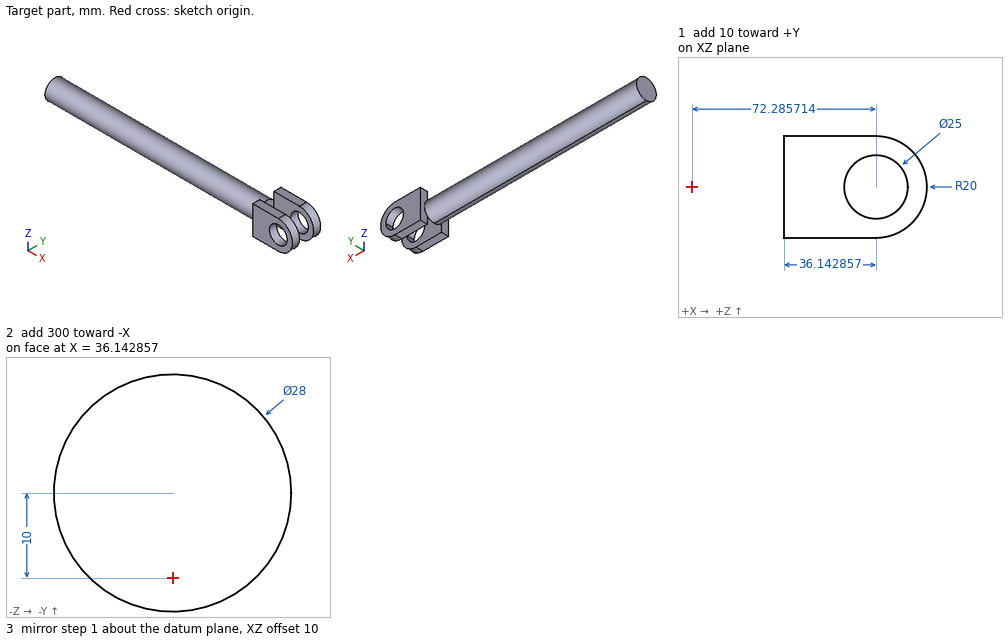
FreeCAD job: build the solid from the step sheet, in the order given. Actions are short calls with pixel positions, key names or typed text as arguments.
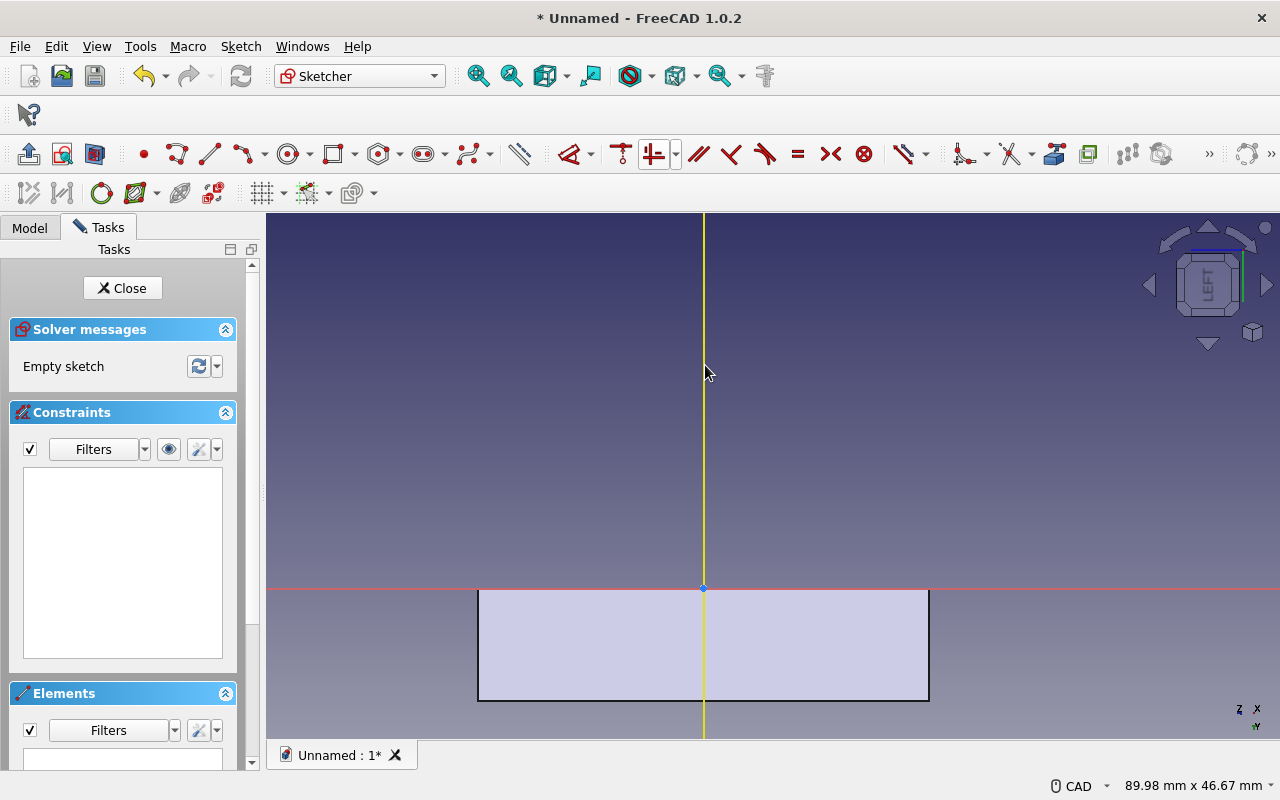
click(288, 154)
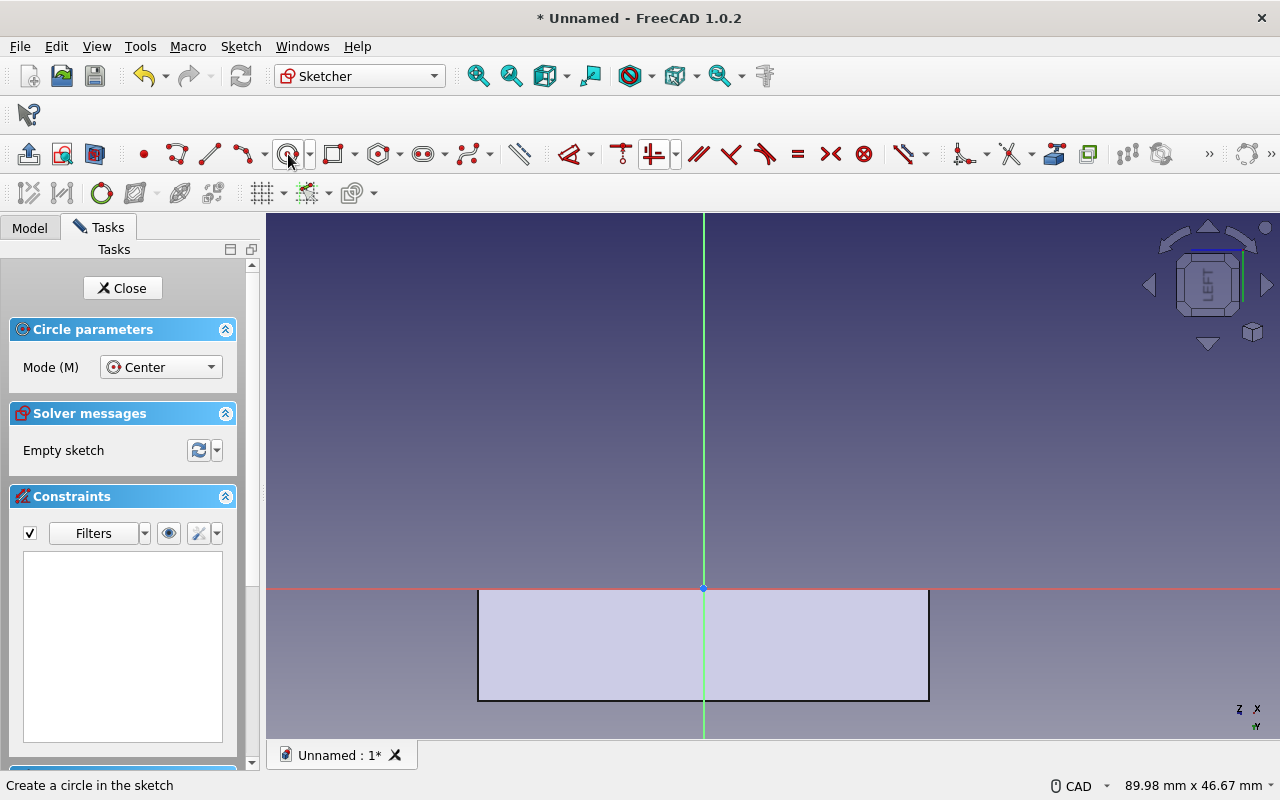
click(704, 476)
move(815, 364)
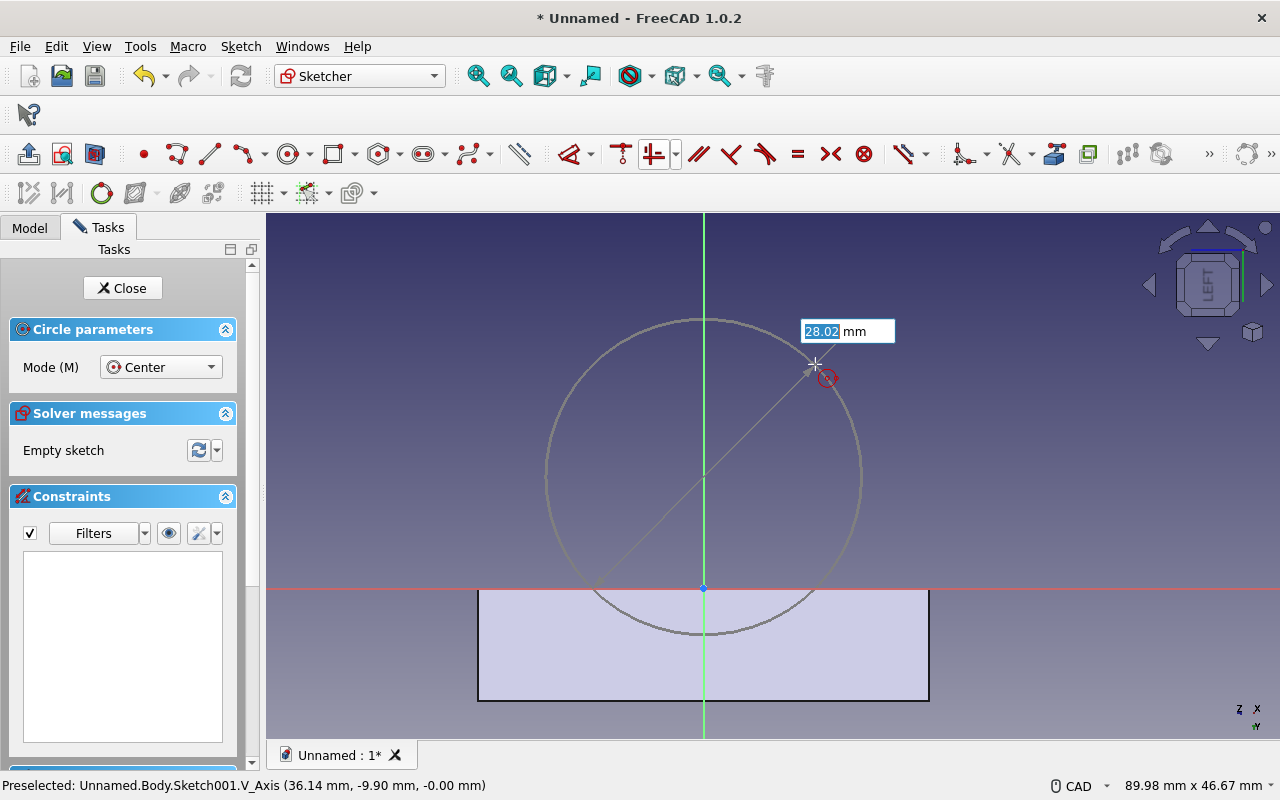
text(28)
key(Return)
key(Escape)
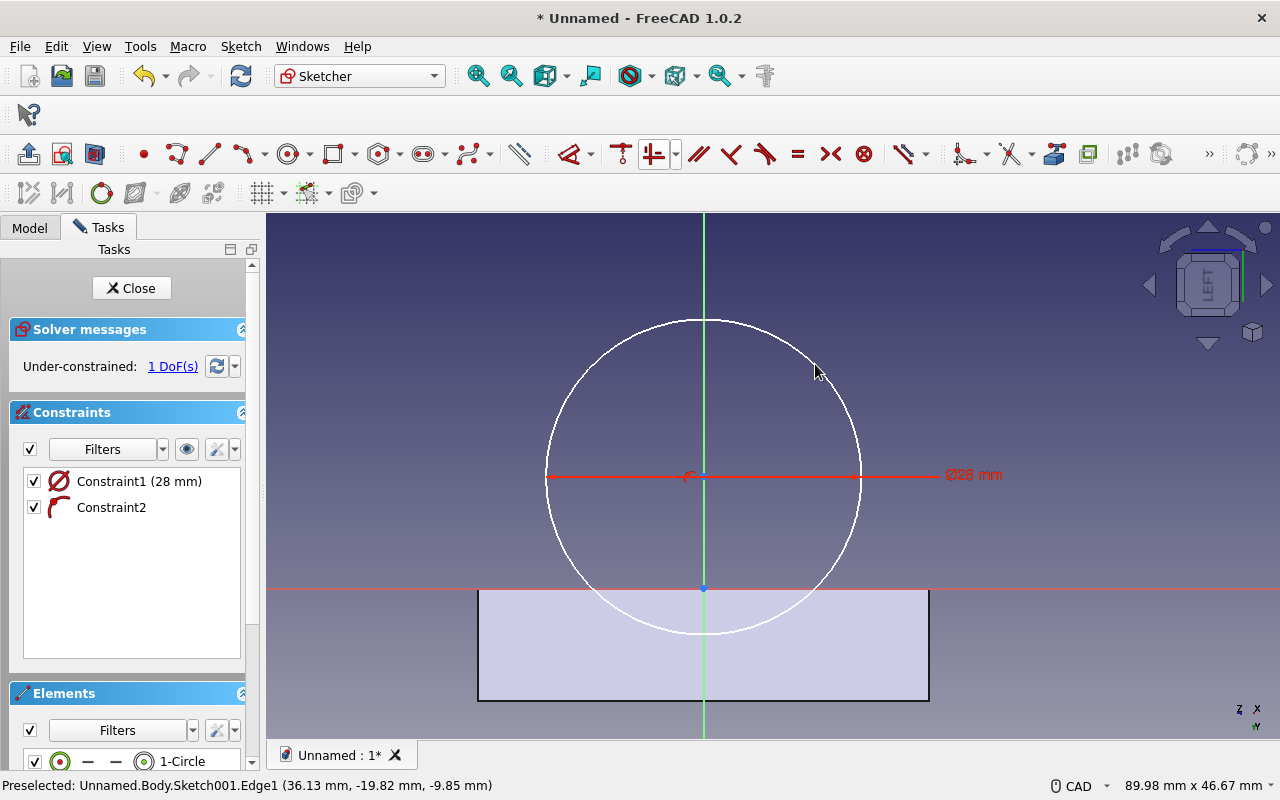
key(d)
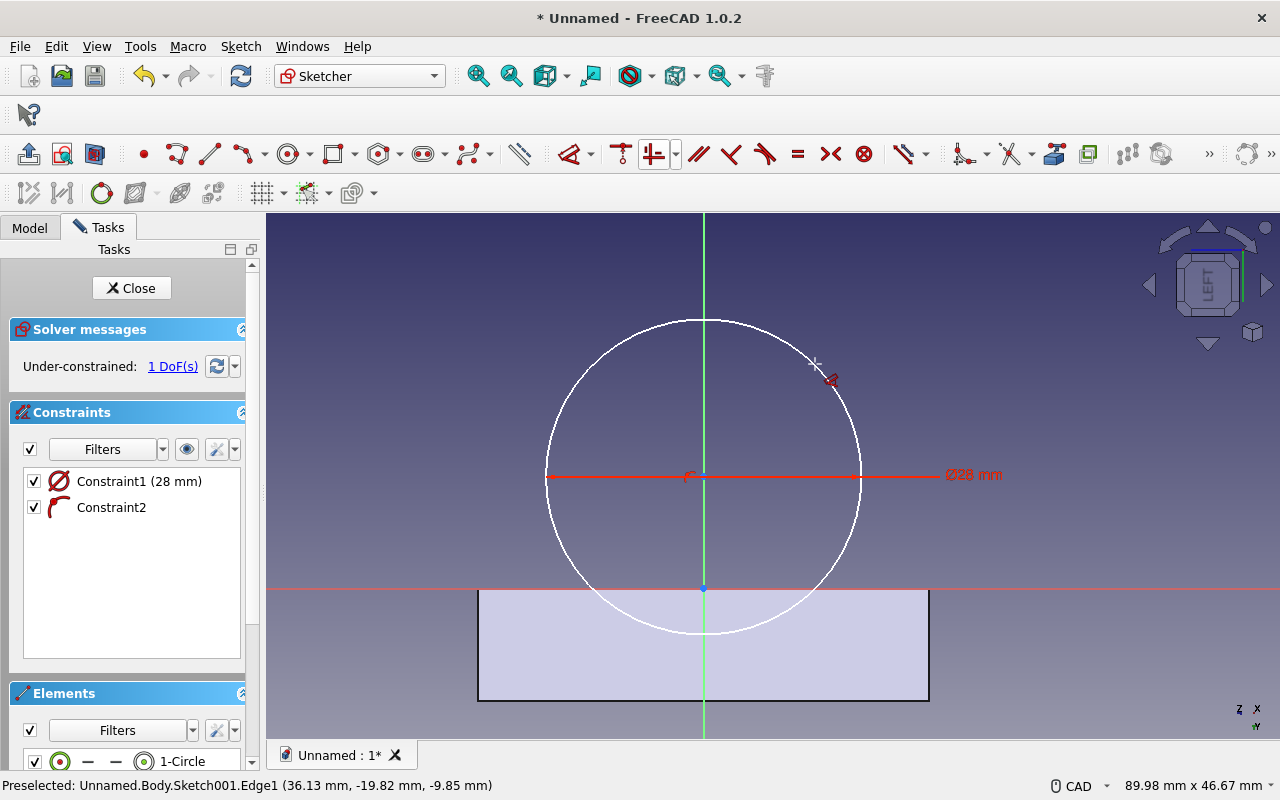
click(704, 477)
click(738, 533)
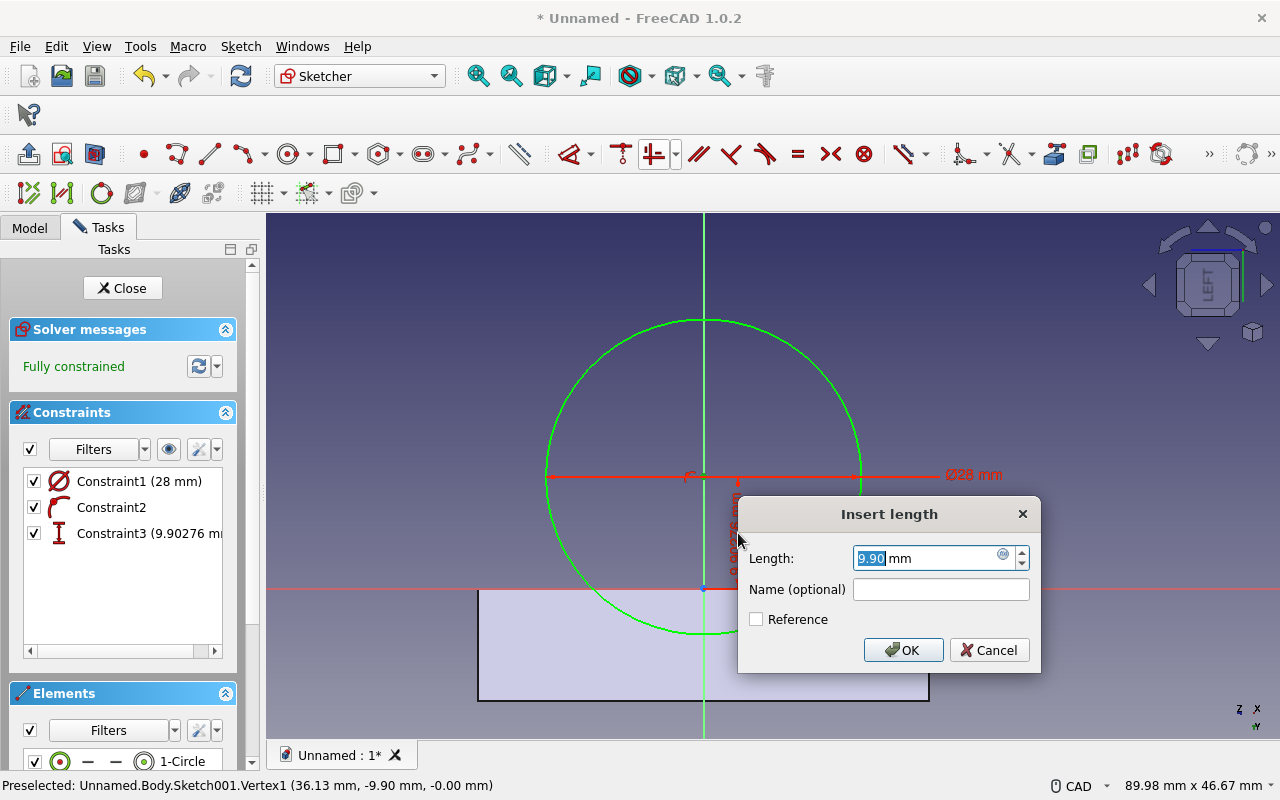
text(10)
key(Return)
key(Escape)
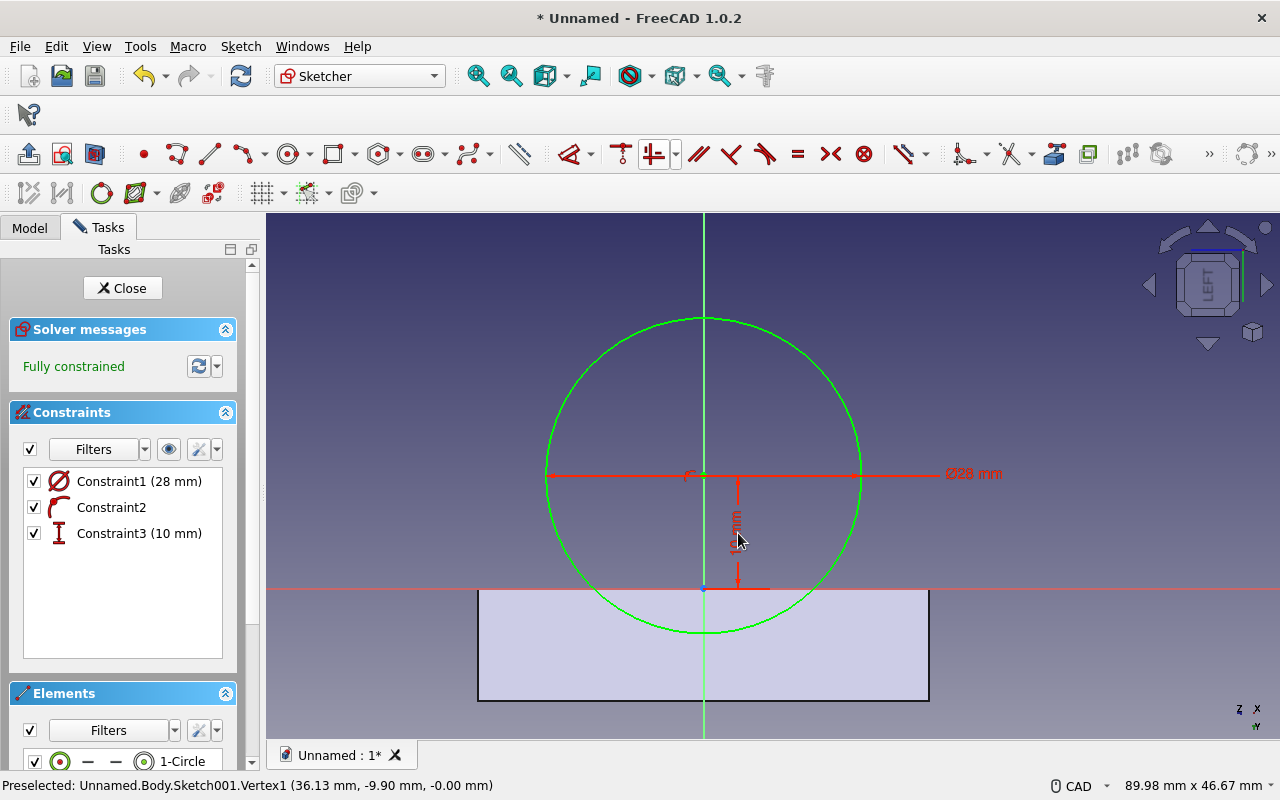
click(123, 288)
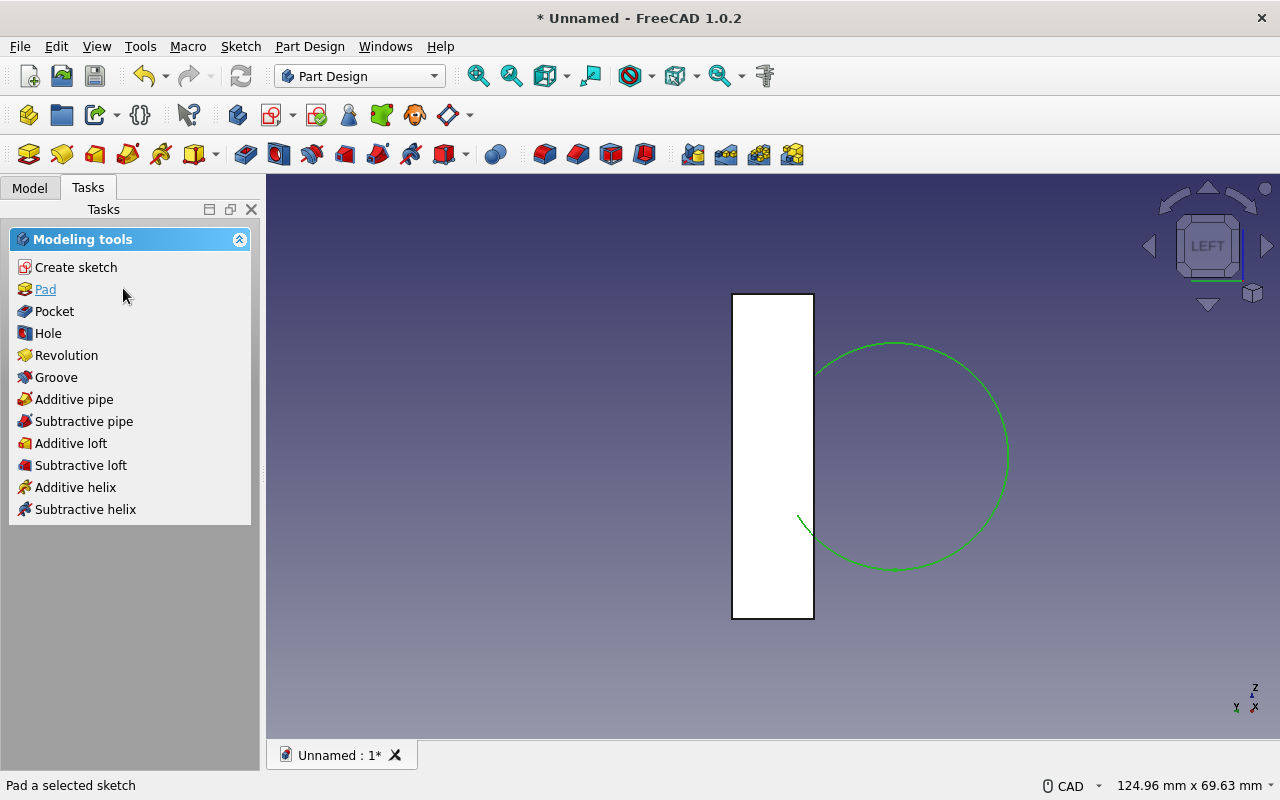
click(29, 154)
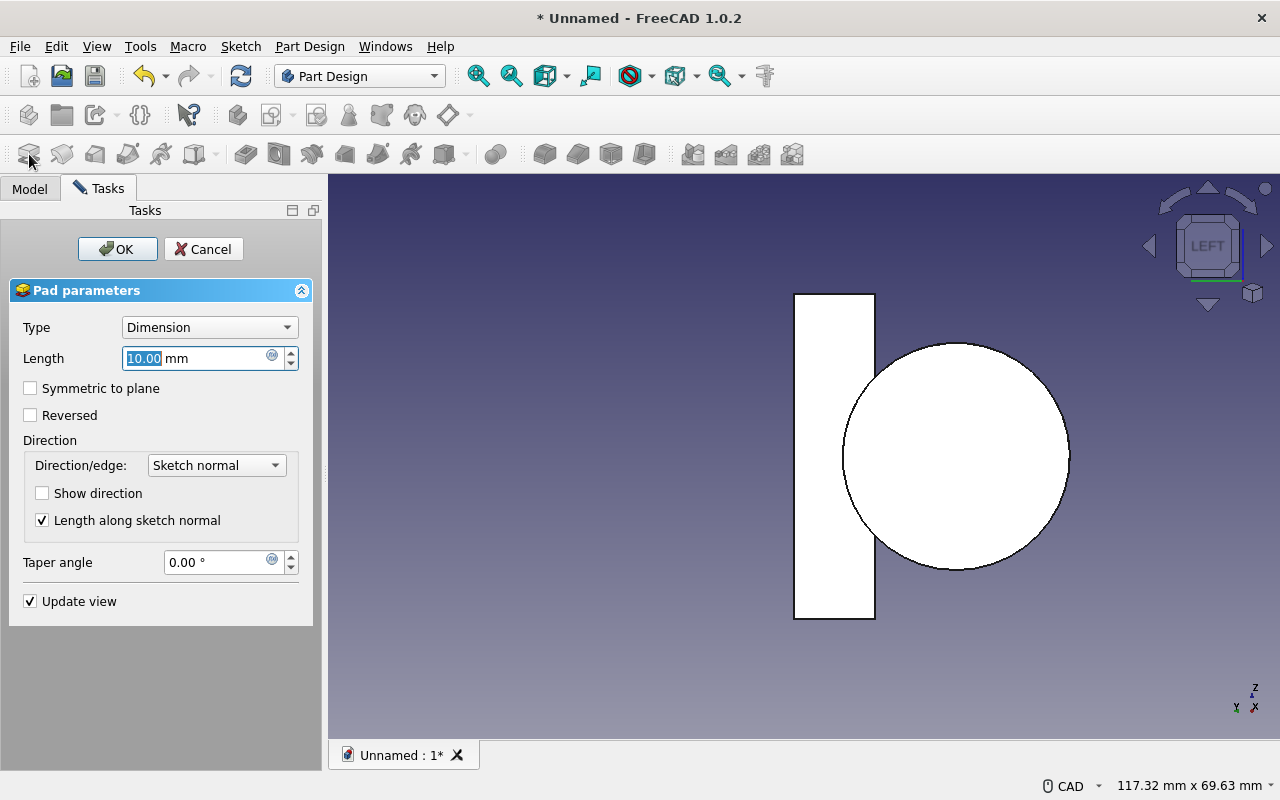
text(300)
key(Tab)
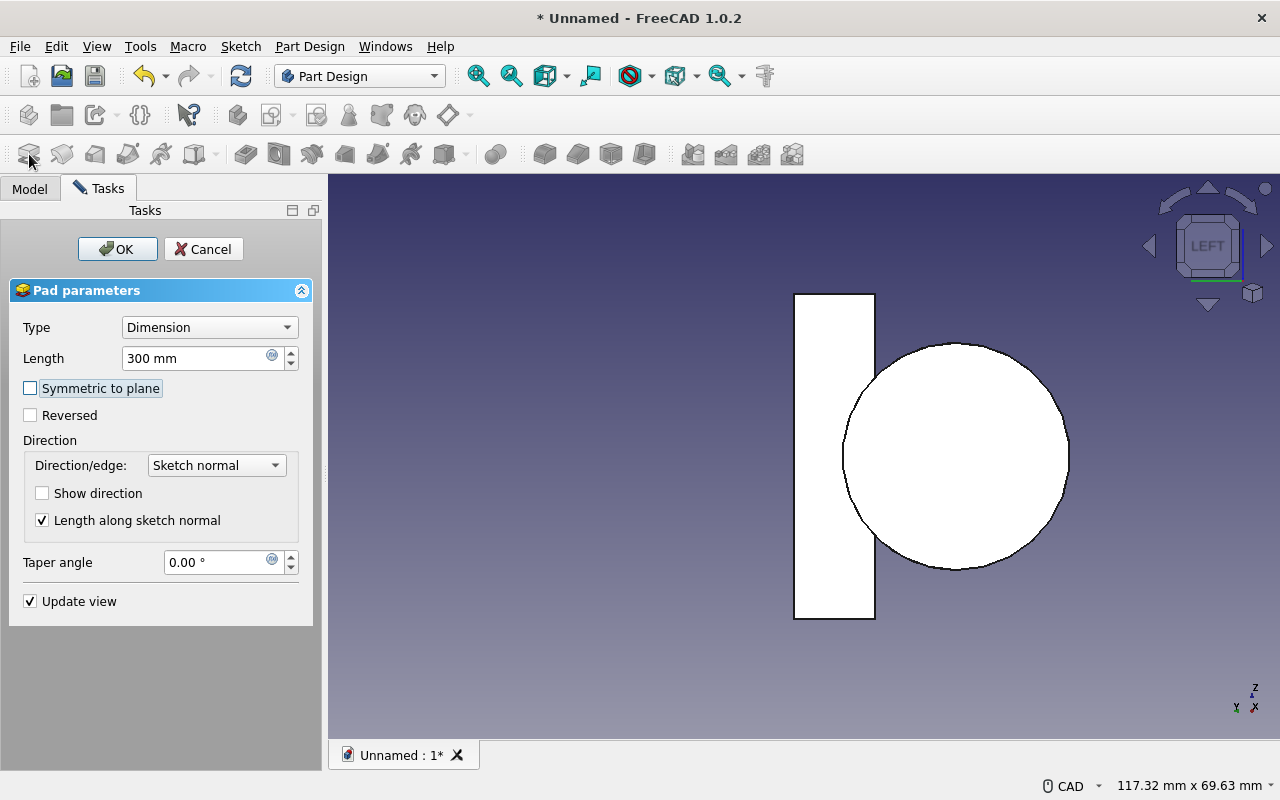
click(118, 249)